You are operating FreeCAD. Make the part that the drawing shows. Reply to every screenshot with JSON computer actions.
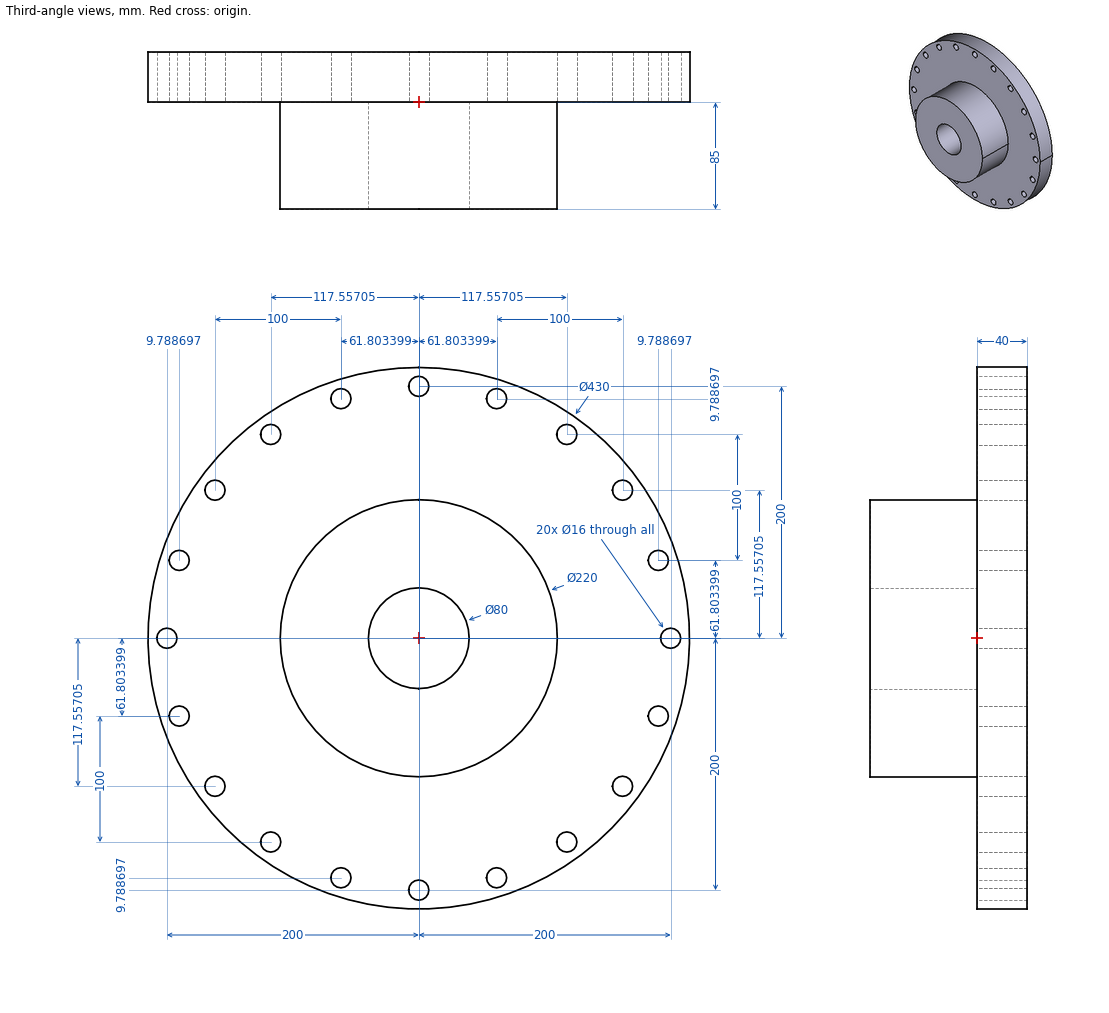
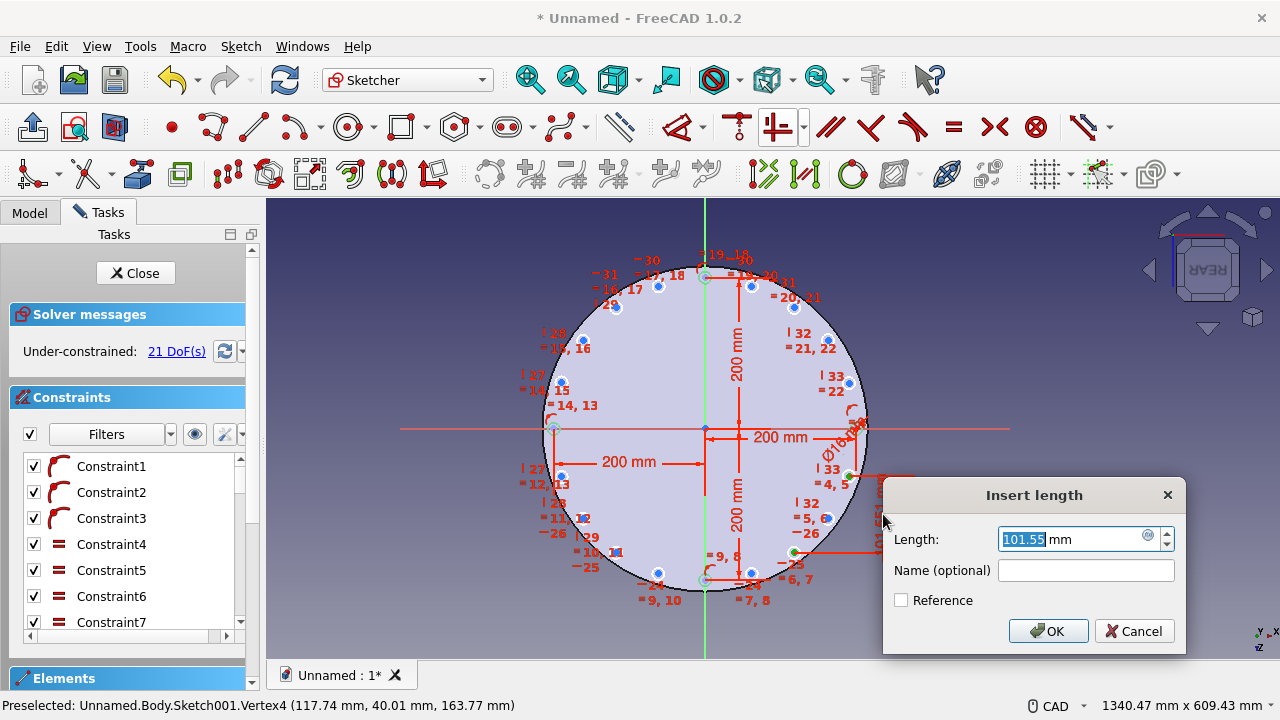
{"action": "type", "text": "100"}
{"action": "key", "text": "Return"}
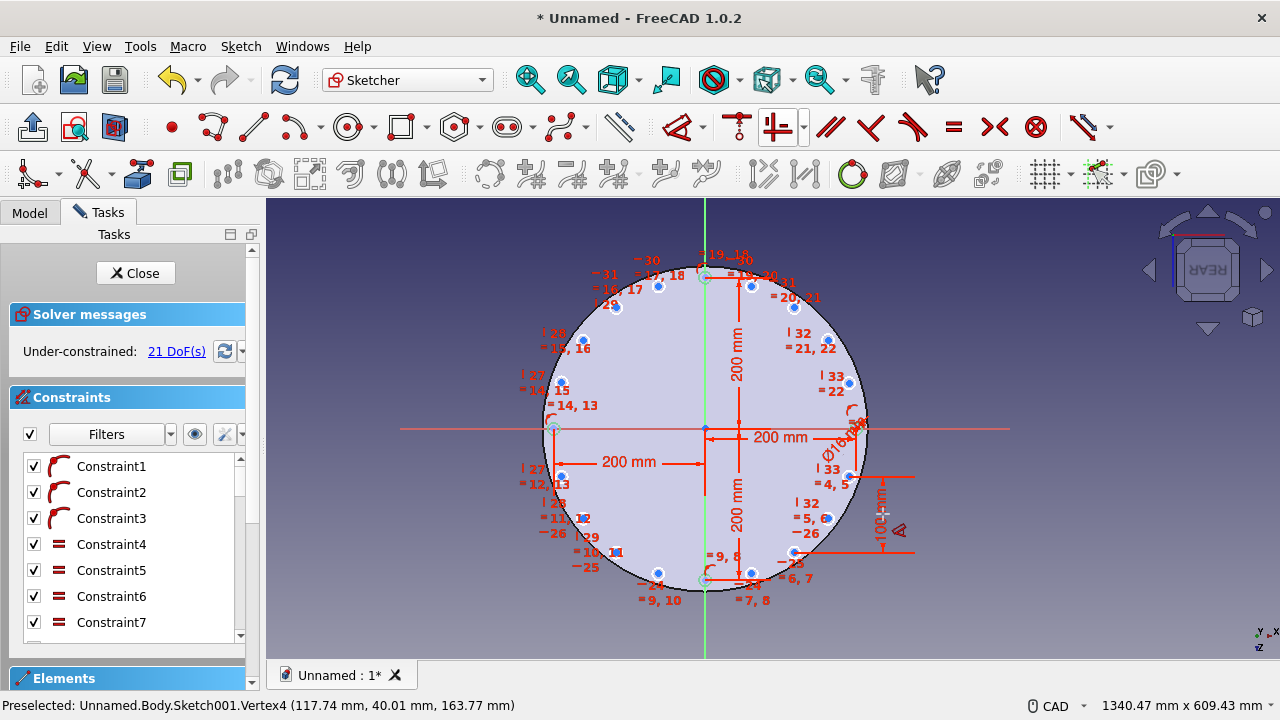
{"action": "left_click", "coordinate": [828, 519]}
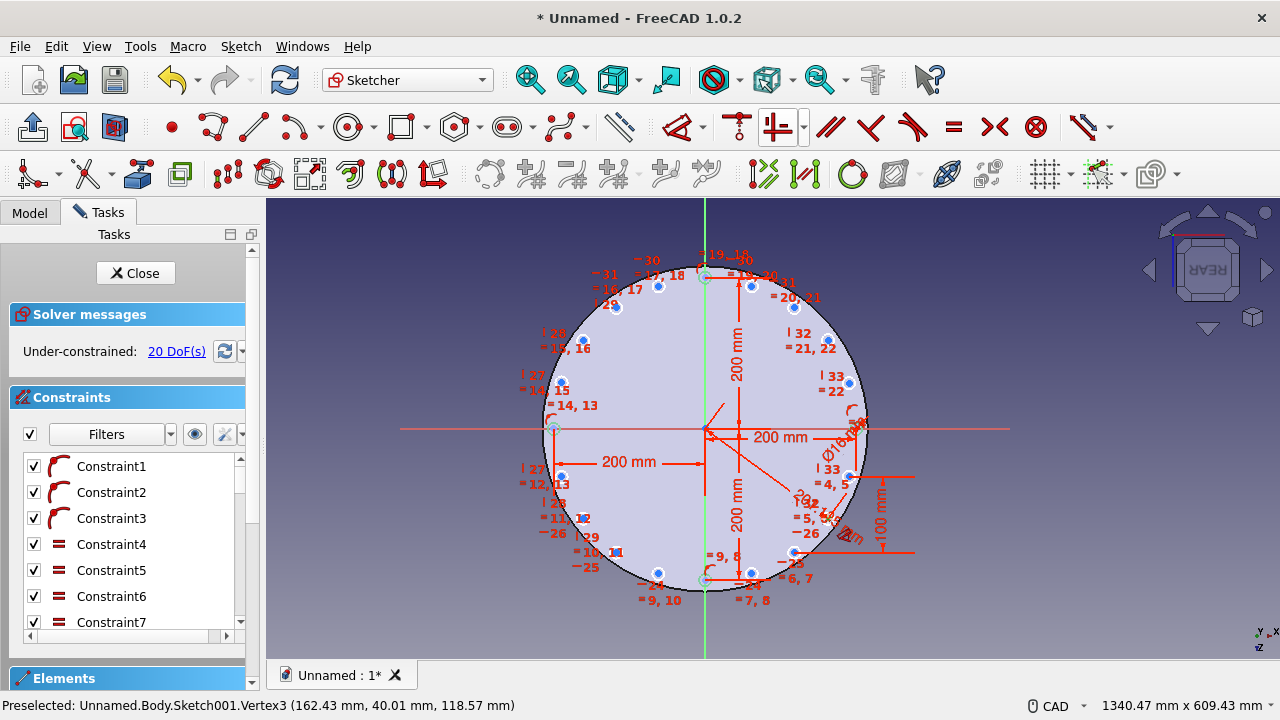
{"action": "left_click", "coordinate": [752, 574]}
{"action": "left_click", "coordinate": [790, 608]}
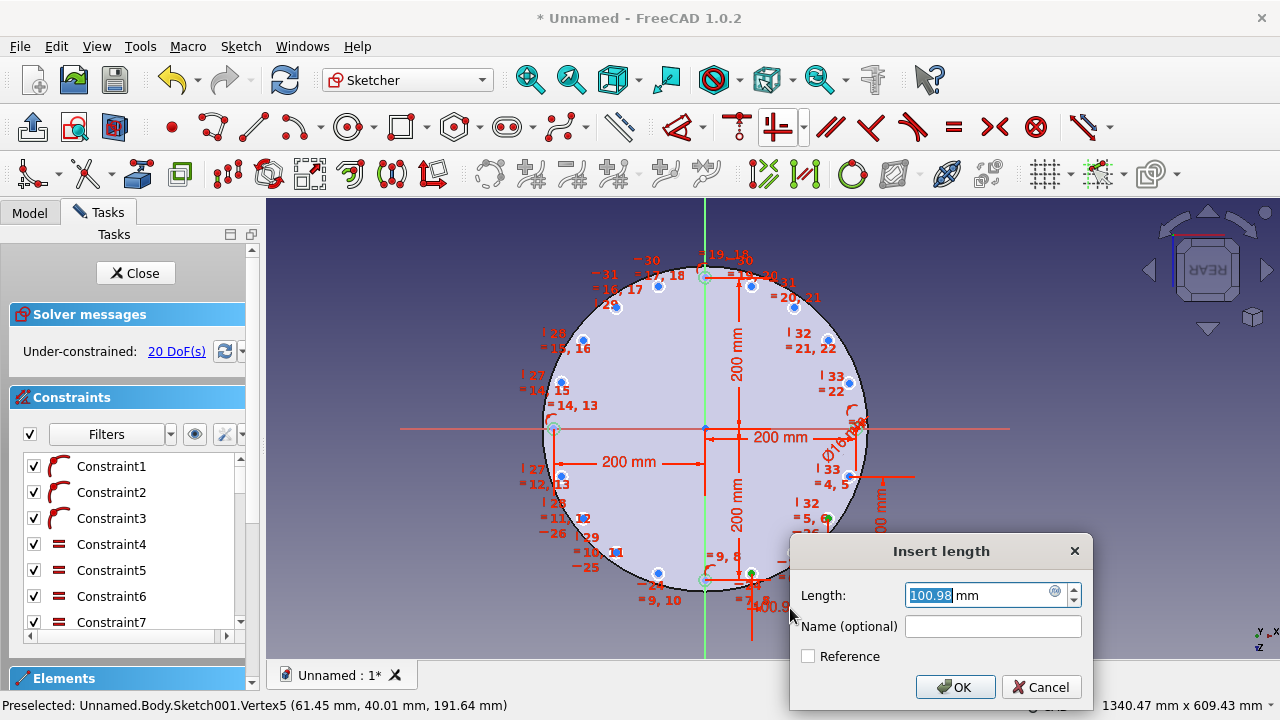
{"action": "type", "text": "100"}
{"action": "key", "text": "Return"}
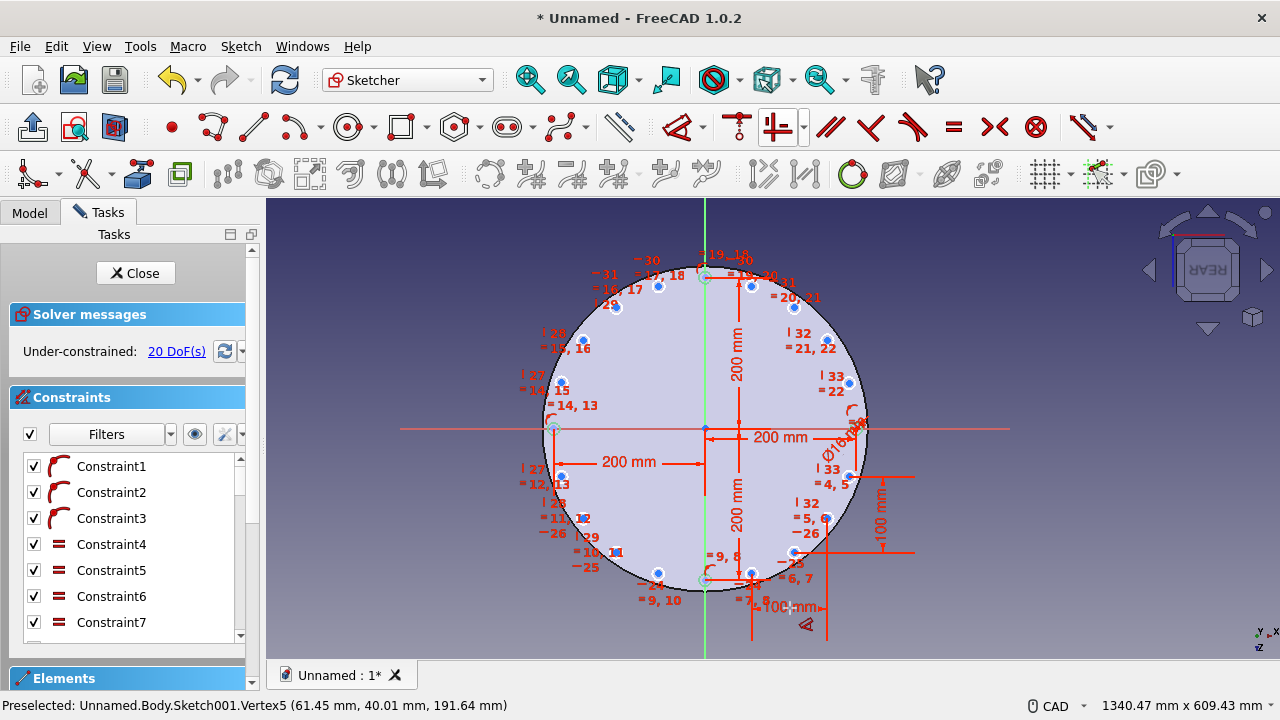
{"action": "left_click", "coordinate": [658, 574]}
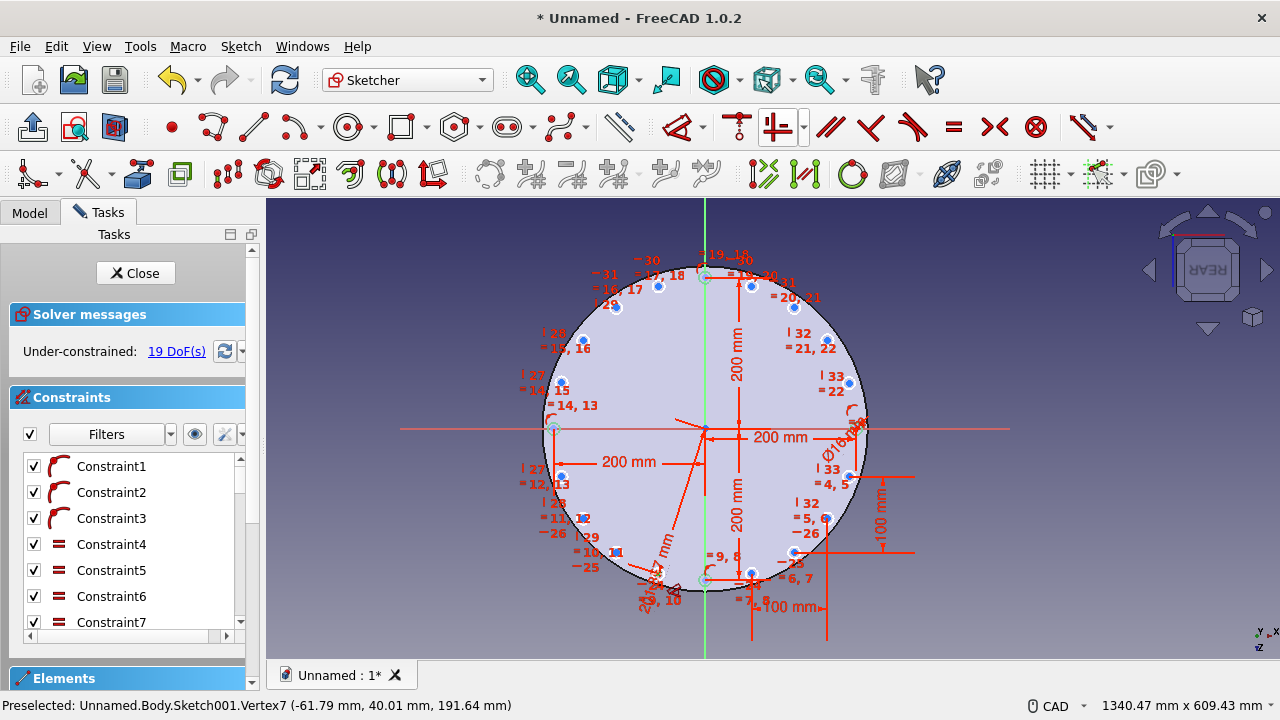
{"action": "left_click", "coordinate": [583, 519]}
{"action": "left_click", "coordinate": [621, 608]}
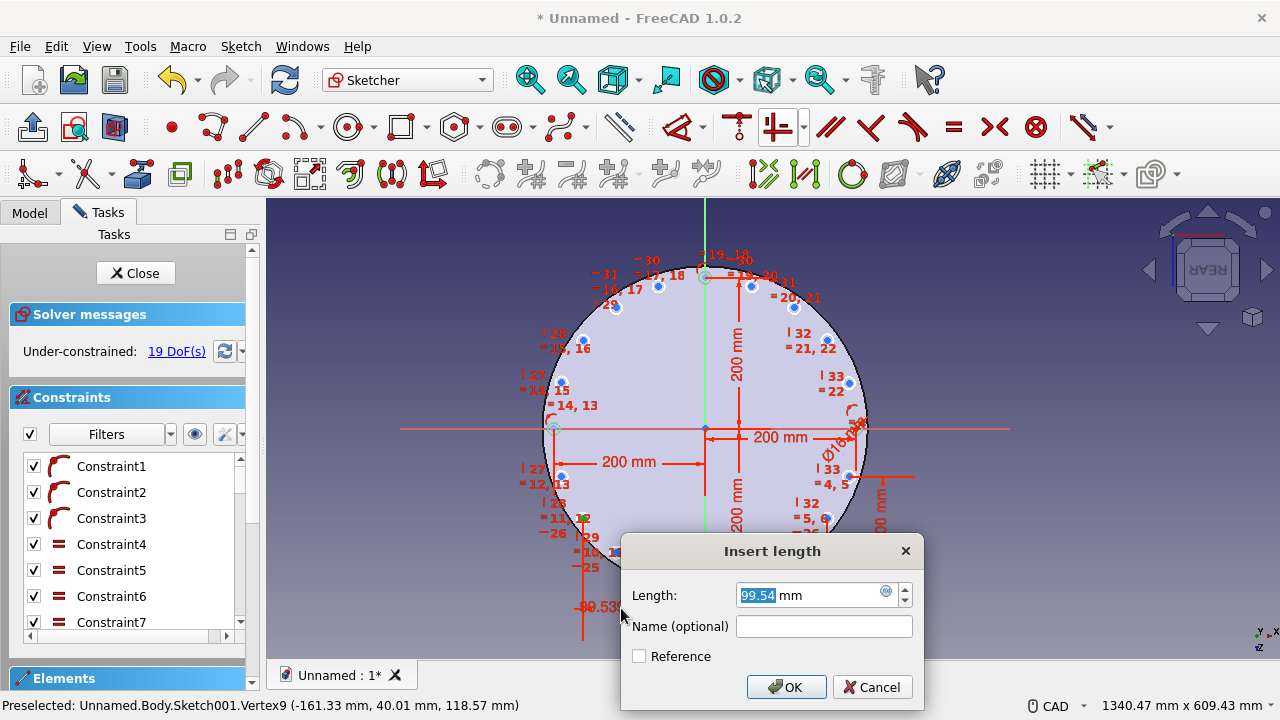
{"action": "type", "text": "100"}
{"action": "key", "text": "Return"}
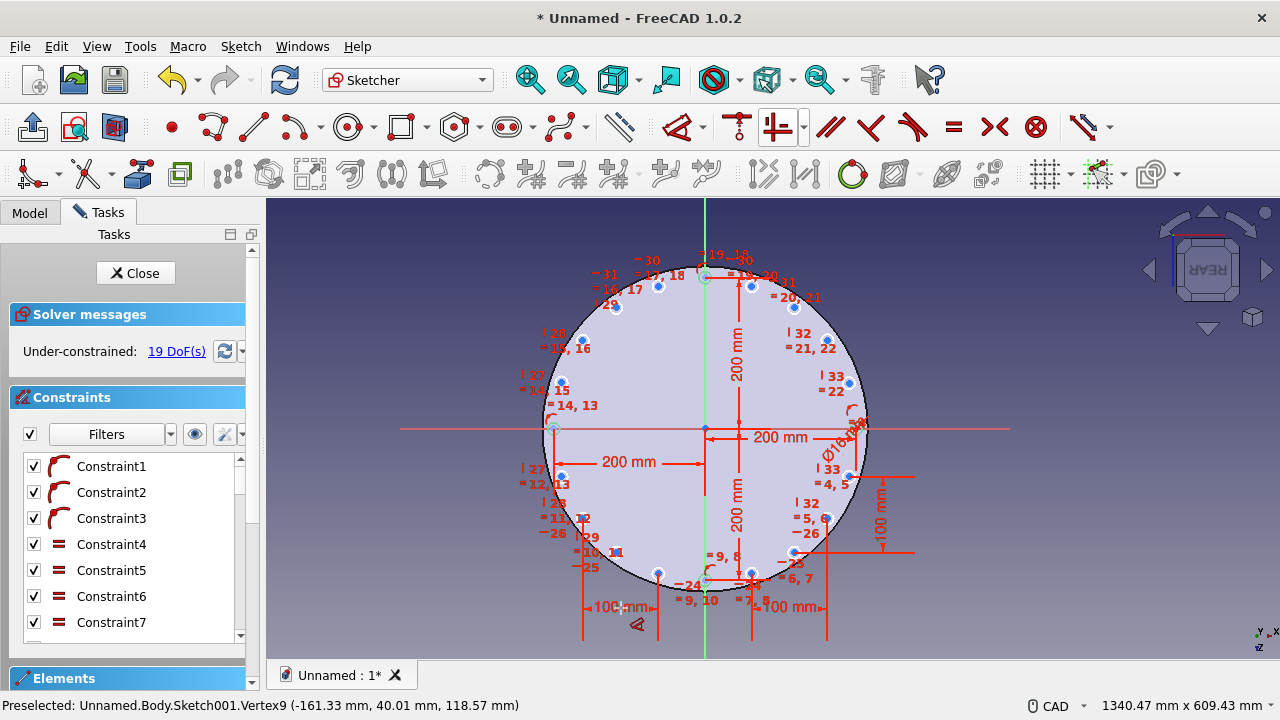
{"action": "left_click", "coordinate": [616, 553]}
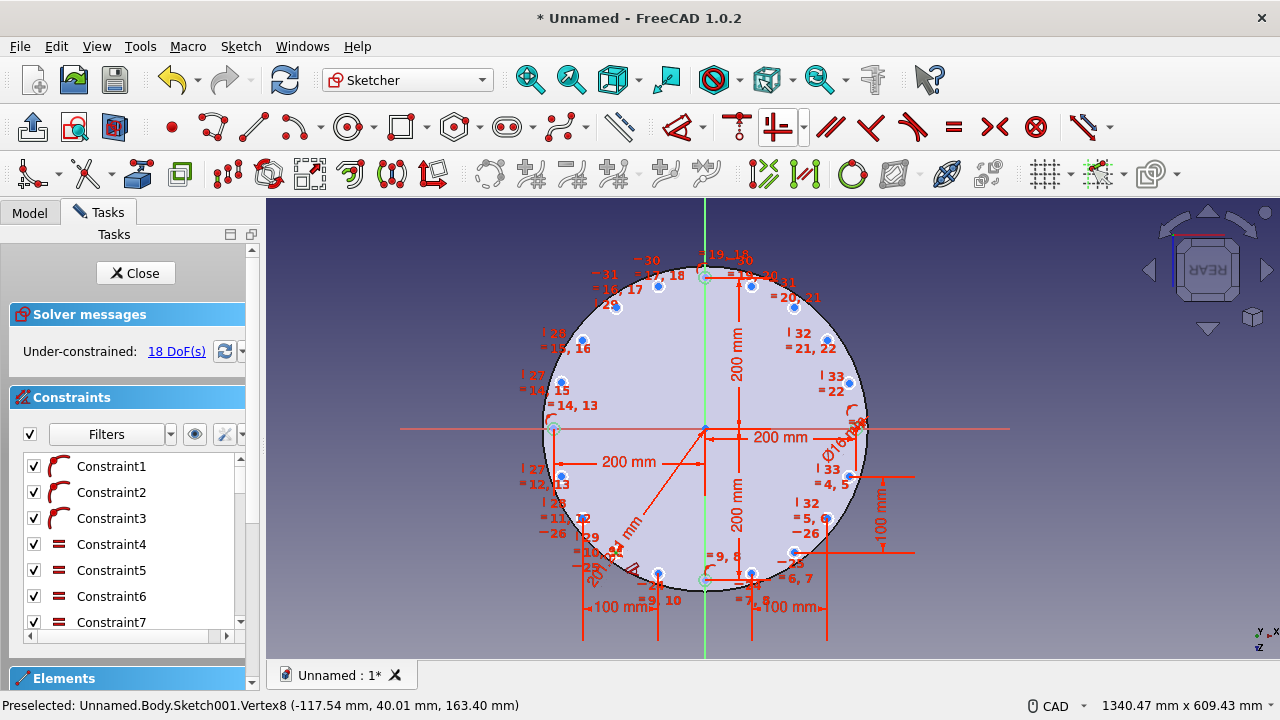
{"action": "left_click", "coordinate": [562, 477]}
{"action": "left_click", "coordinate": [528, 515]}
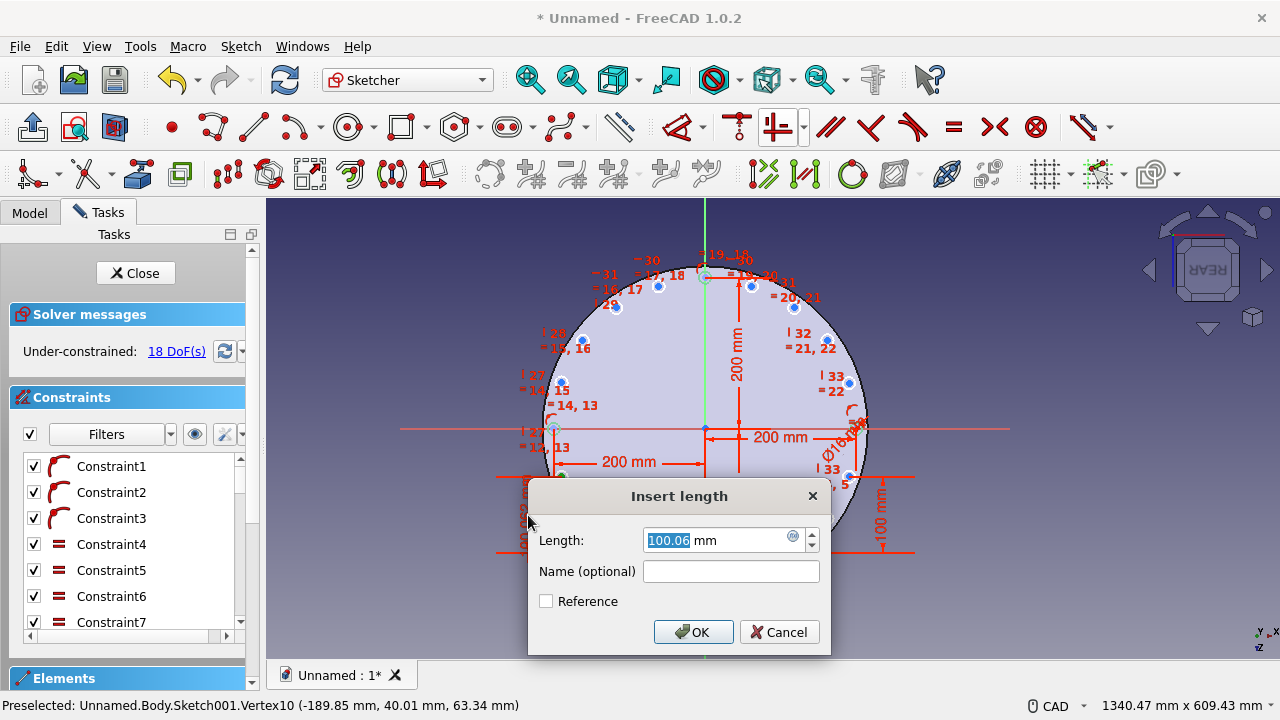
{"action": "type", "text": "100"}
{"action": "key", "text": "Return"}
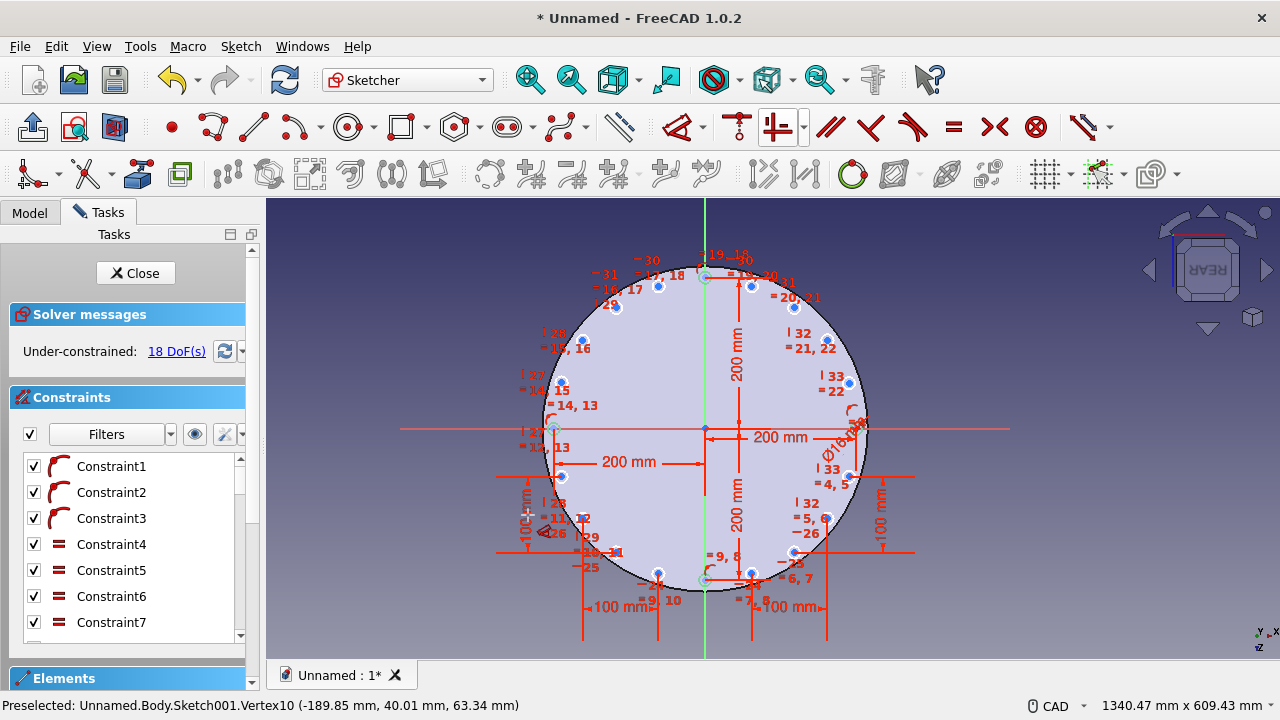
{"action": "left_click", "coordinate": [562, 383]}